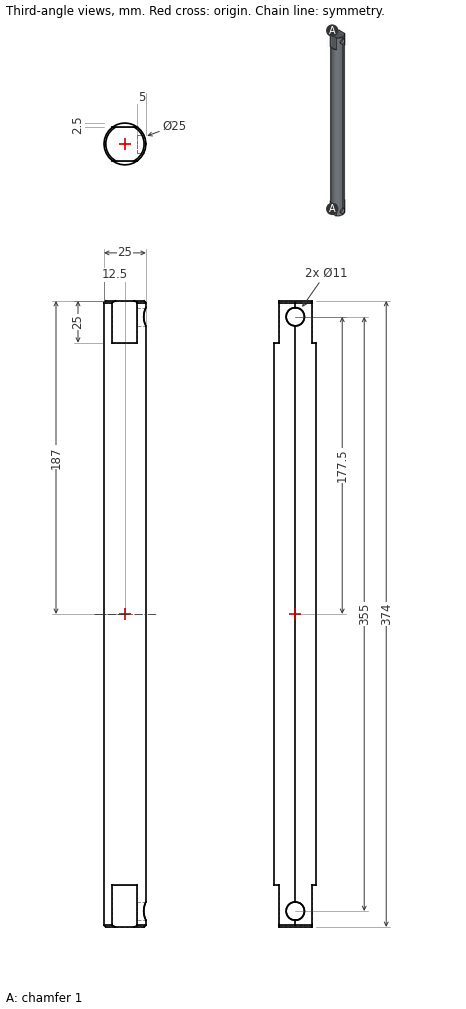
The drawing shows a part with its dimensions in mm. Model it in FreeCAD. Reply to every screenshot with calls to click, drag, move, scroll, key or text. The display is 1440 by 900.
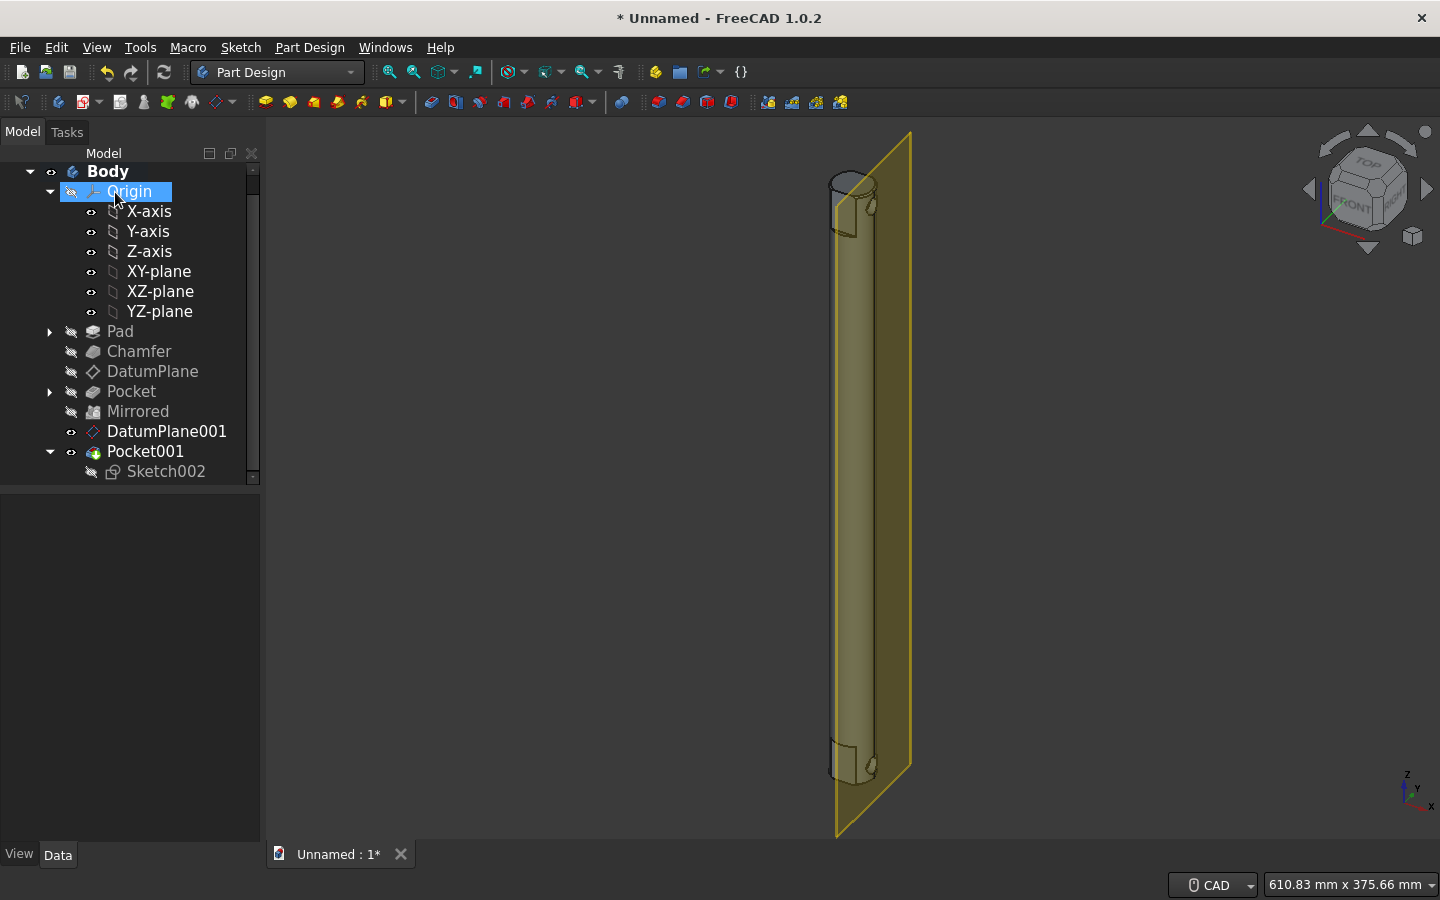
click(116, 432)
key(space)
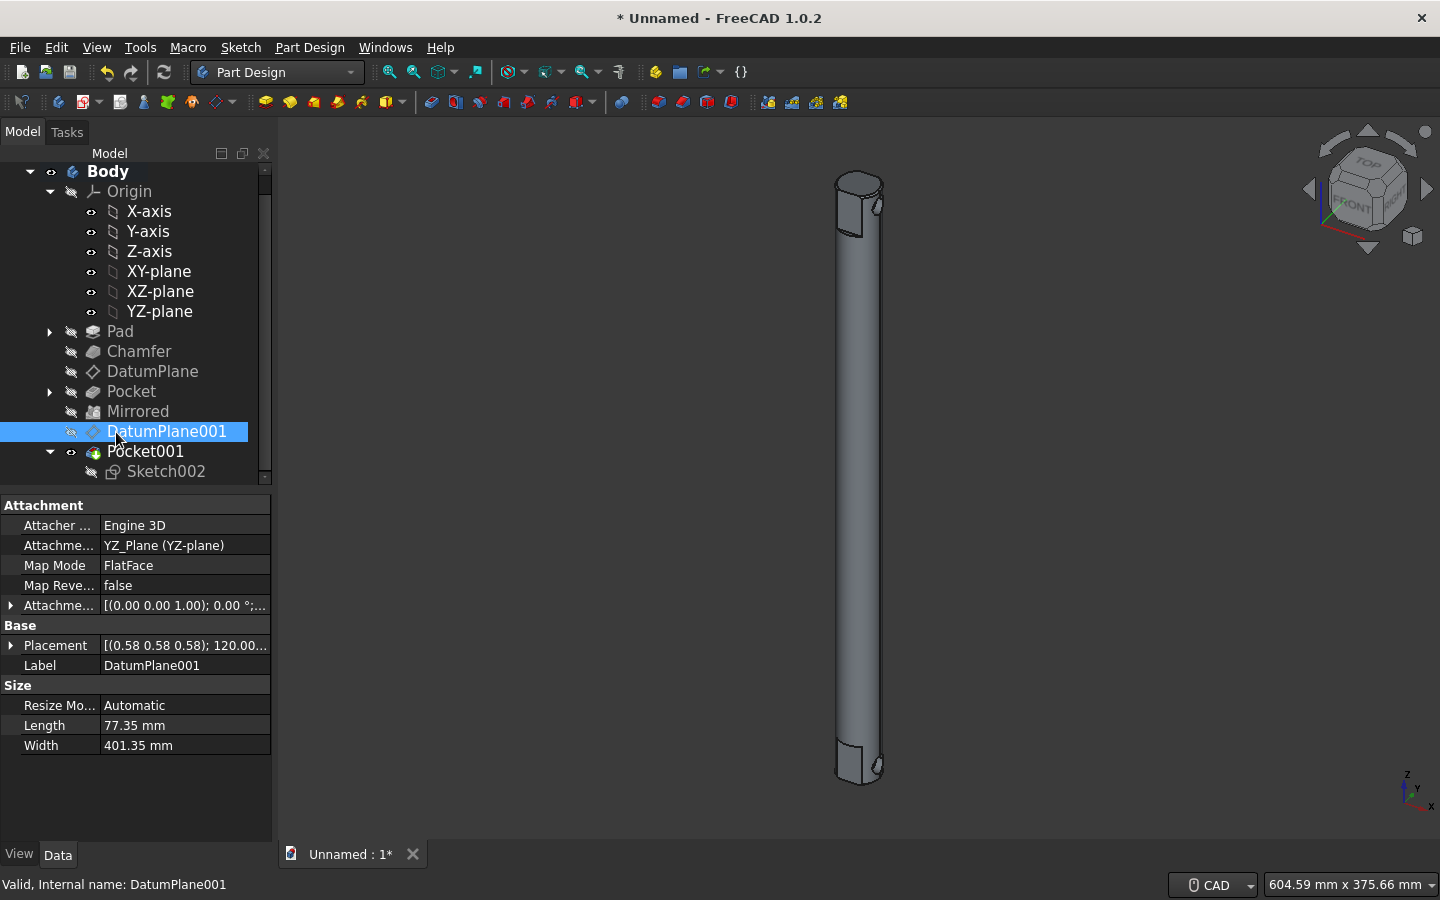
key(0)